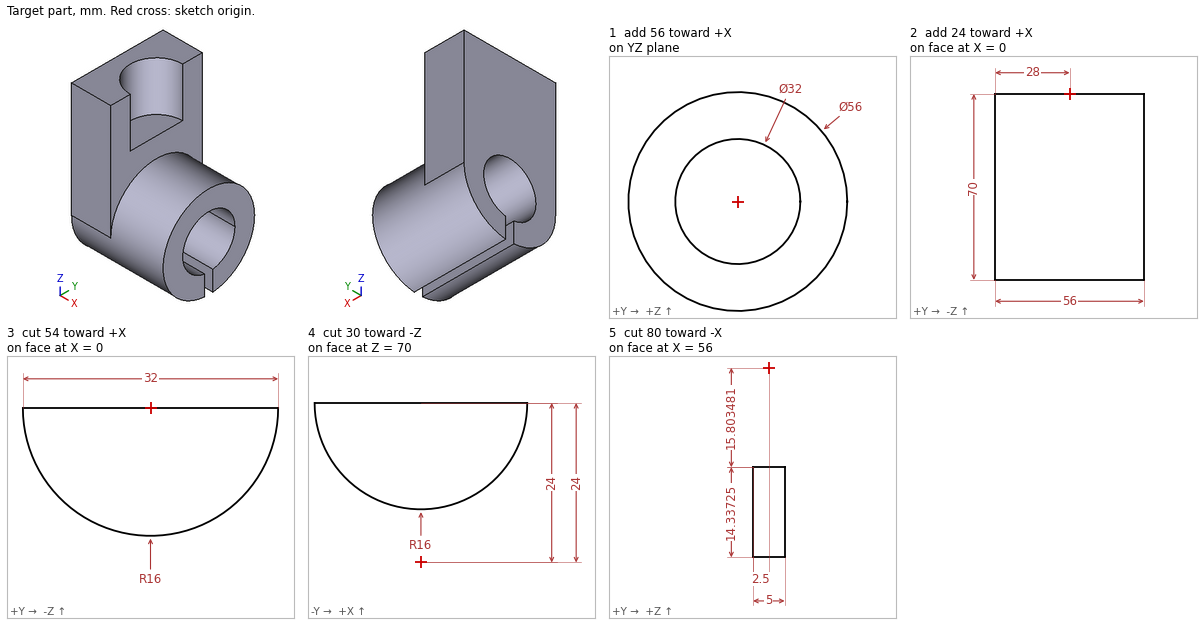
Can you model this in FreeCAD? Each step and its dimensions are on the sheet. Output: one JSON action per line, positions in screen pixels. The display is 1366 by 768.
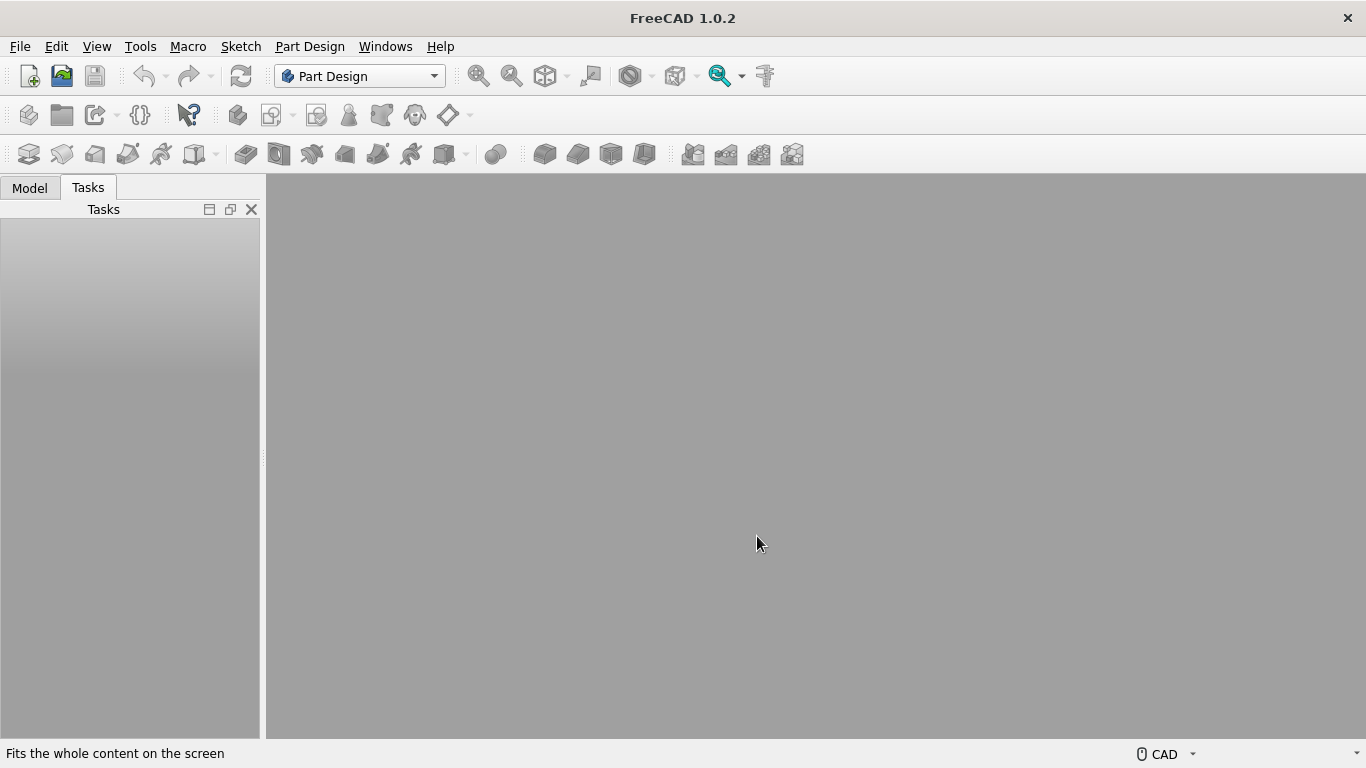
{"action": "left_click", "coordinate": [29, 76]}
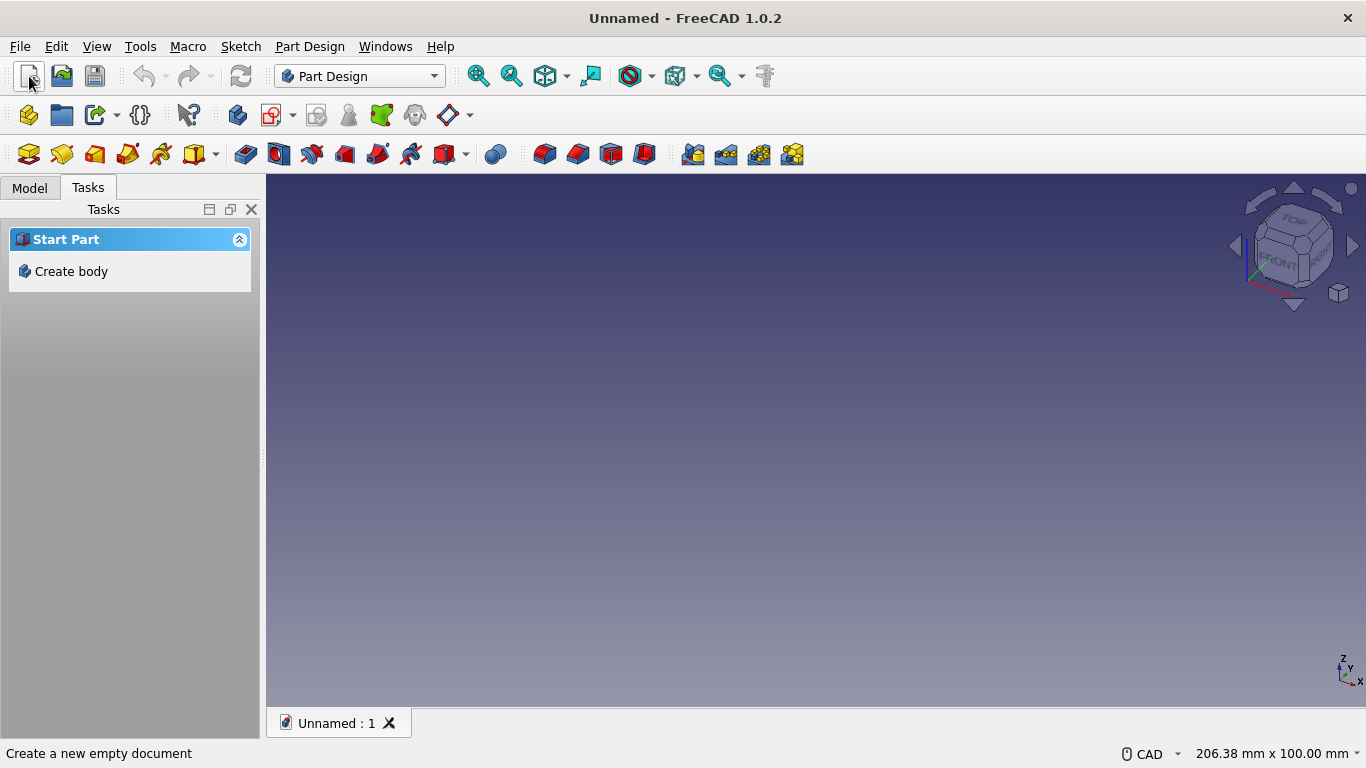
{"action": "left_click", "coordinate": [270, 116]}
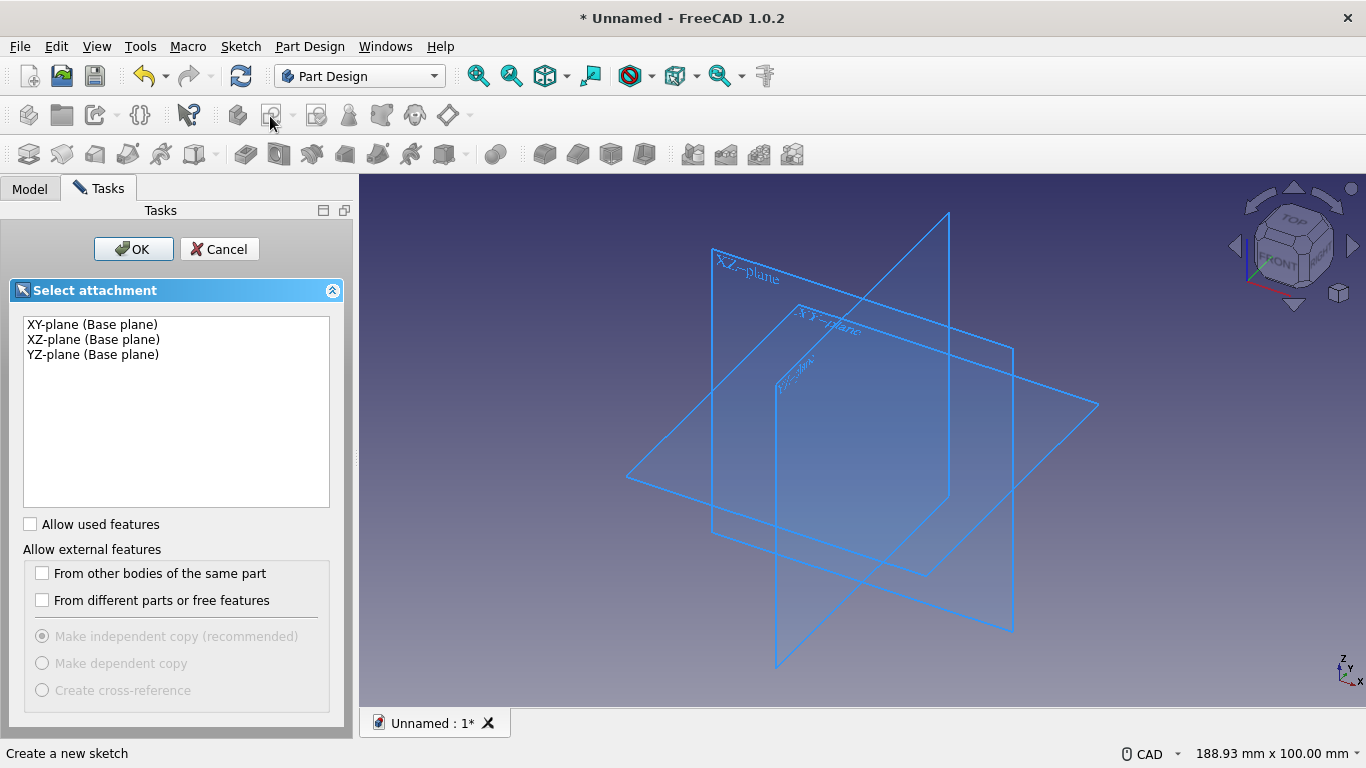
{"action": "left_click", "coordinate": [84, 354]}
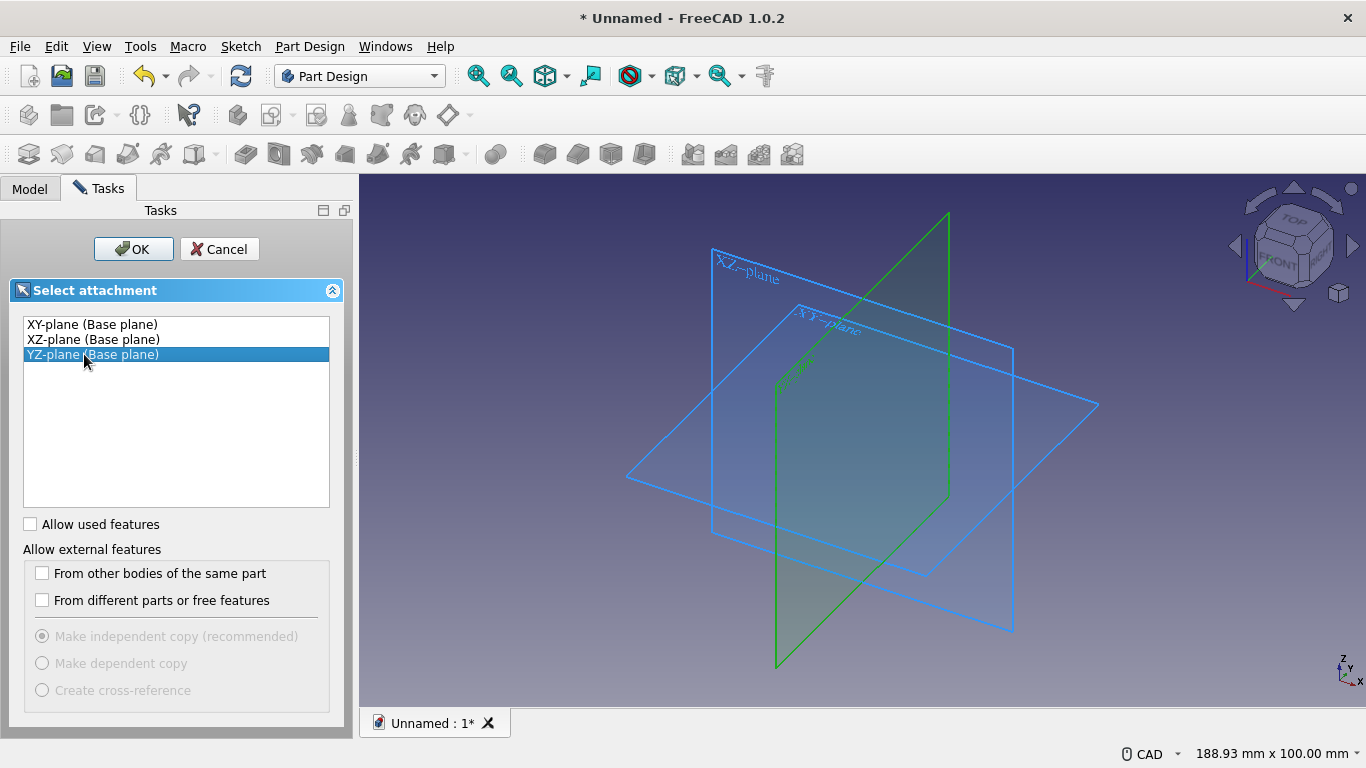
{"action": "left_click", "coordinate": [134, 249]}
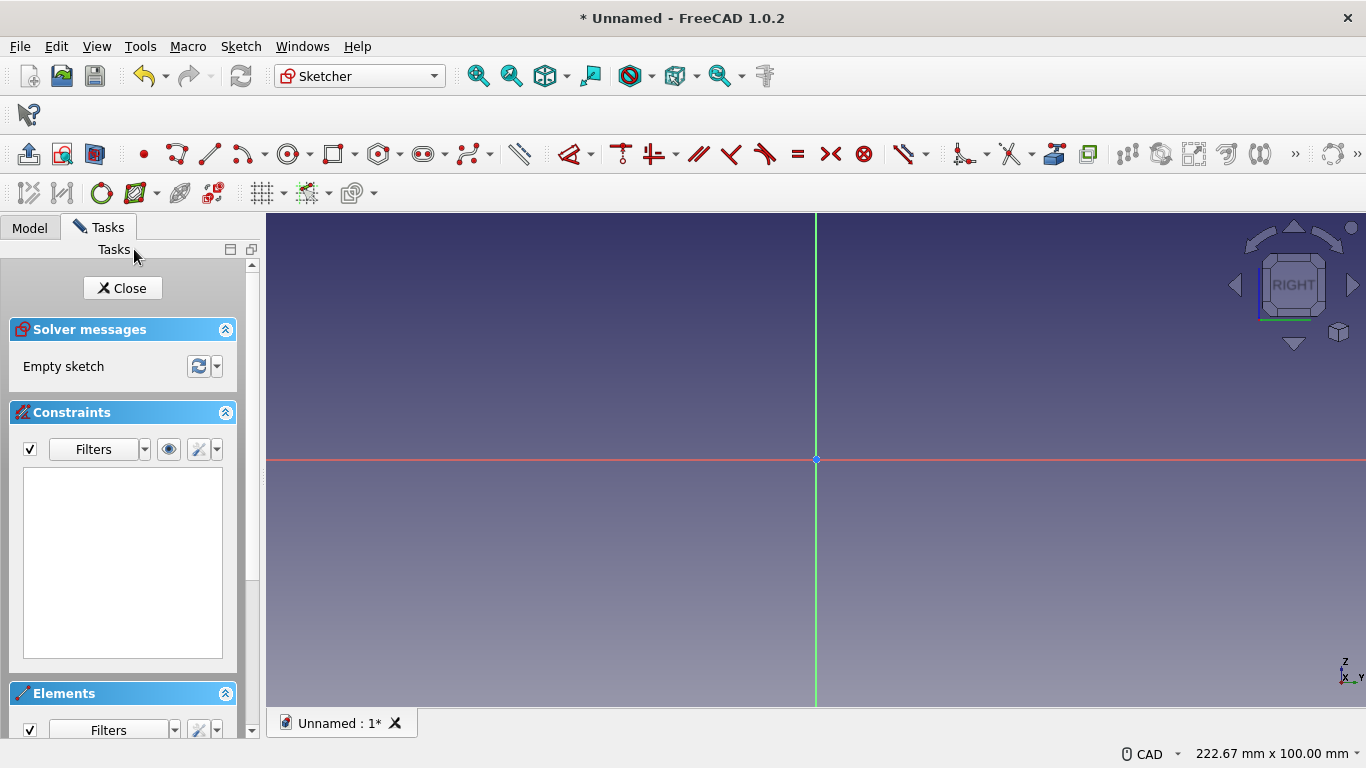
{"action": "key", "text": "g c"}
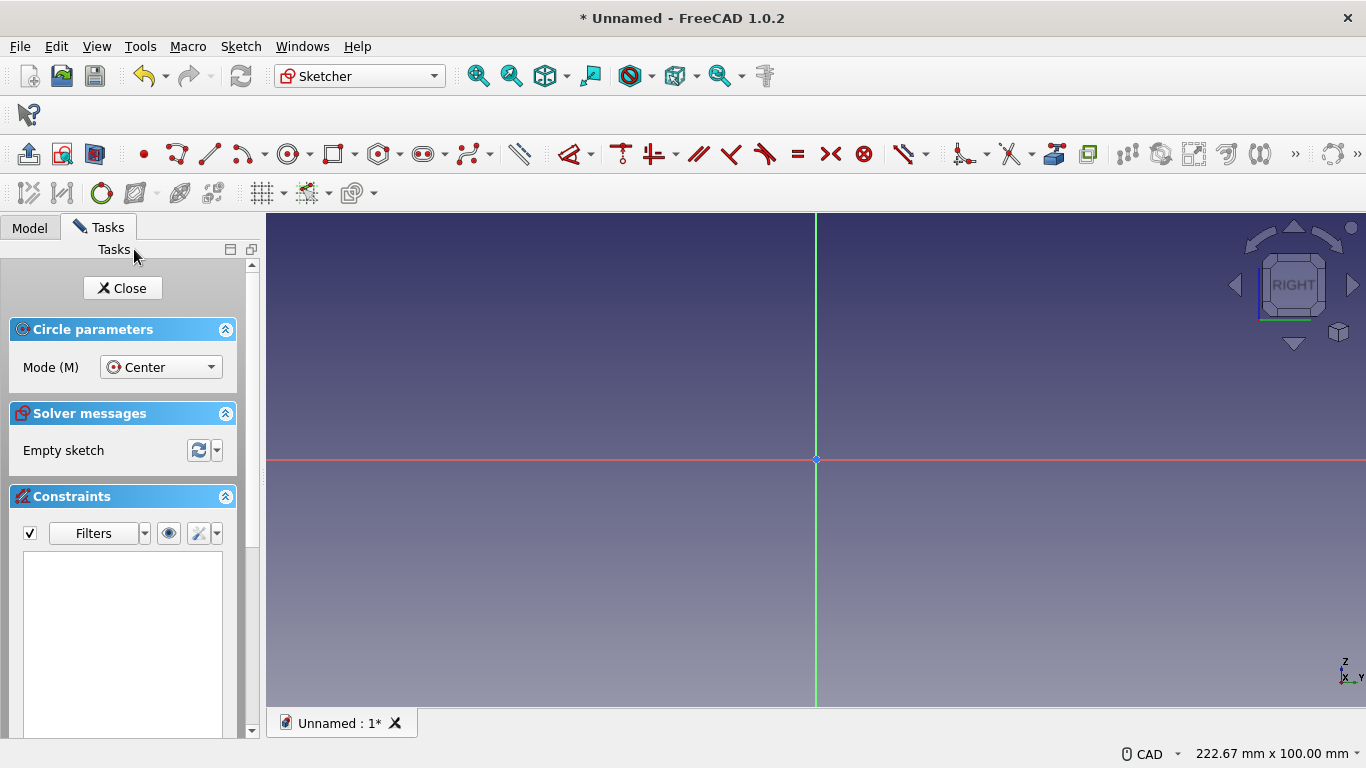
{"action": "left_click", "coordinate": [816, 460]}
{"action": "left_click", "coordinate": [914, 362]}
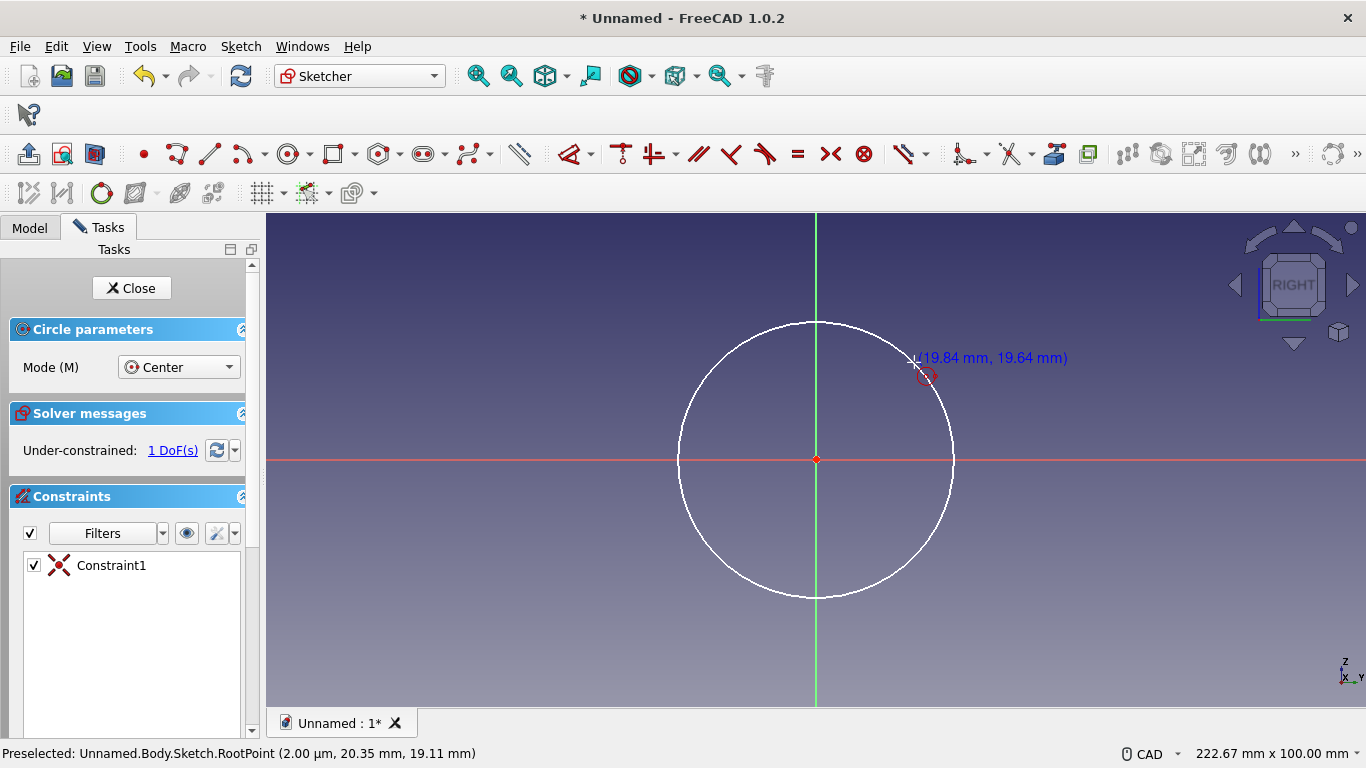
{"action": "left_click", "coordinate": [816, 460]}
{"action": "left_click", "coordinate": [872, 404]}
{"action": "key", "text": "Escape"}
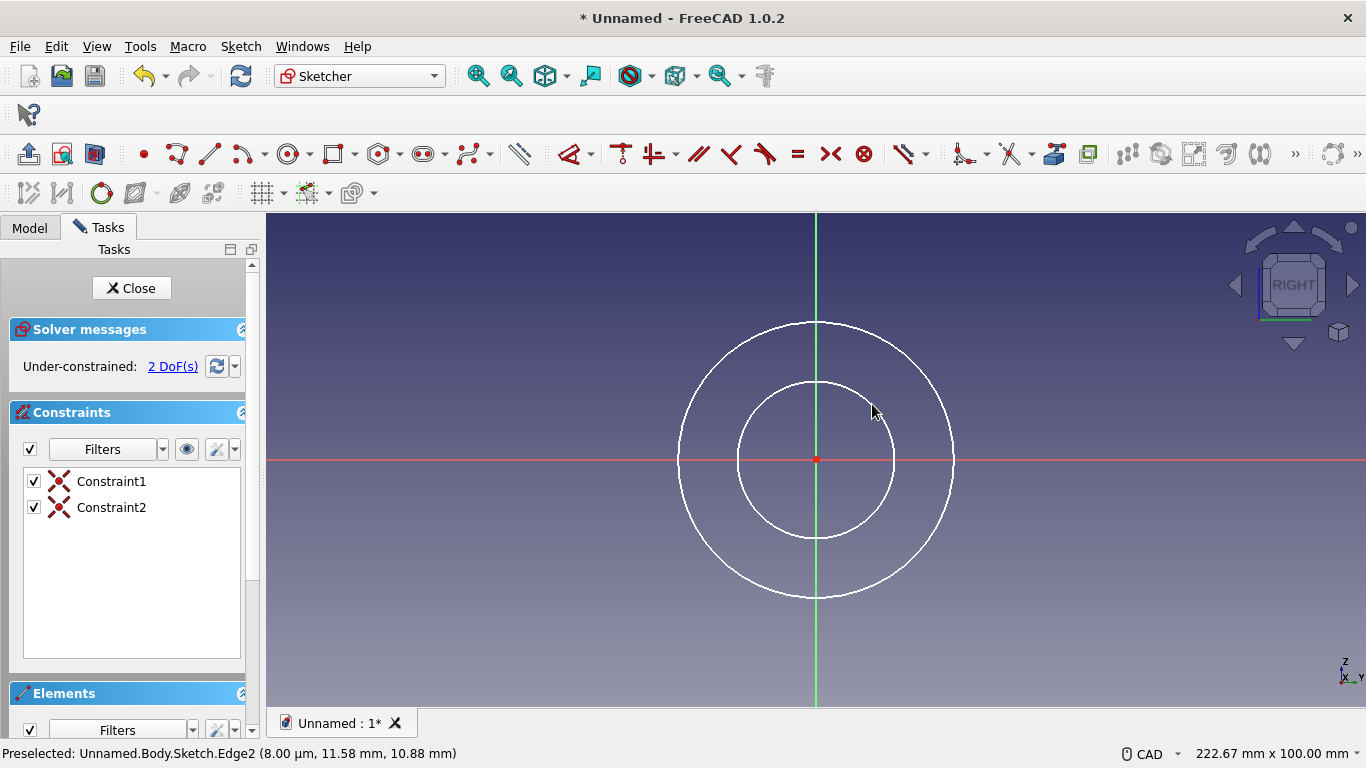
{"action": "left_click", "coordinate": [913, 362]}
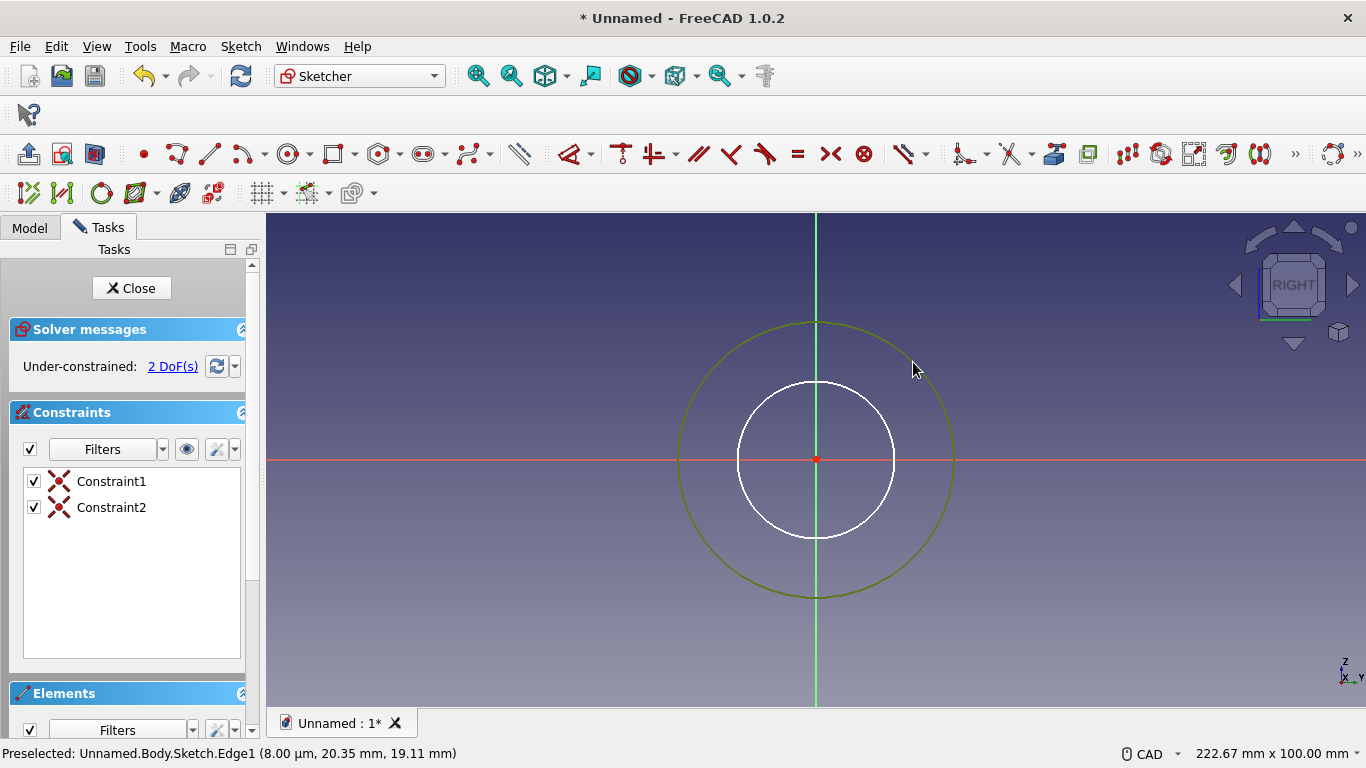
{"action": "key", "text": "k o"}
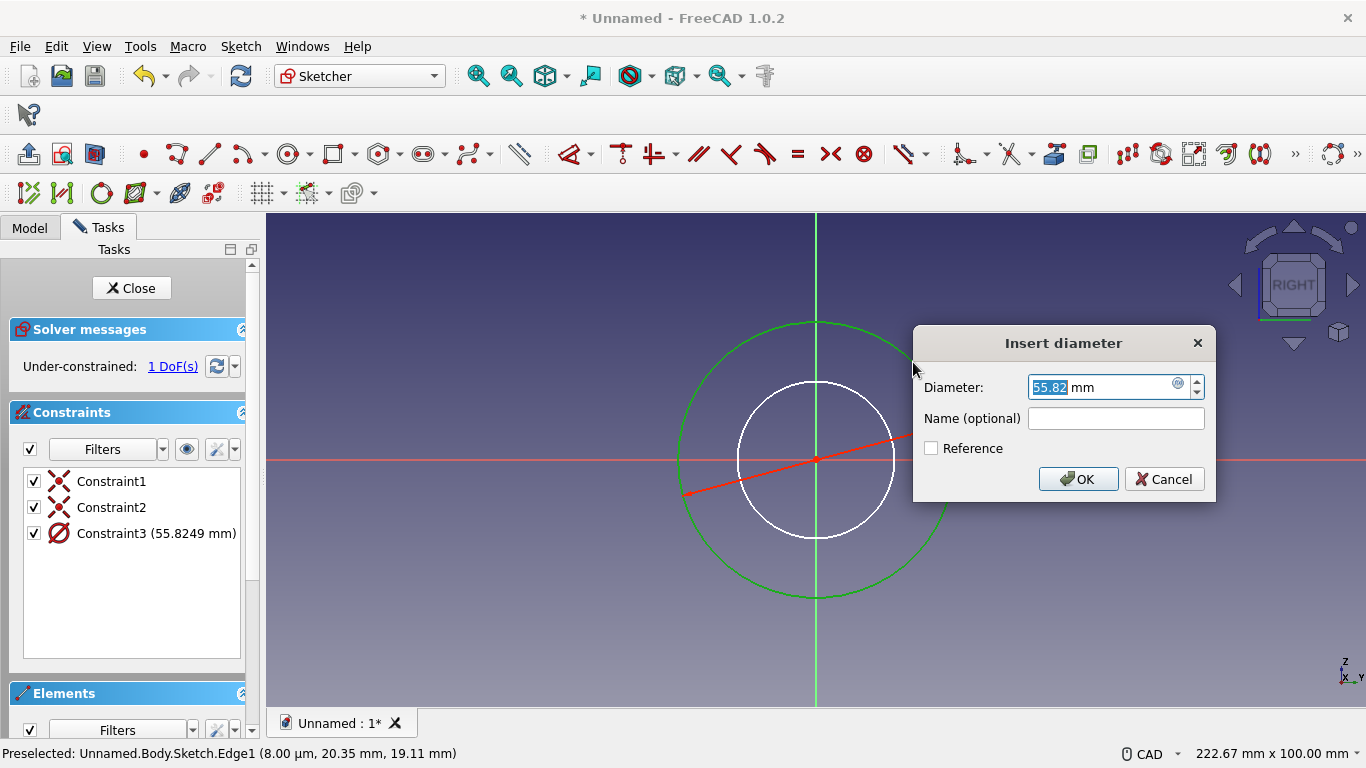
{"action": "type", "text": "56"}
{"action": "key", "text": "Return"}